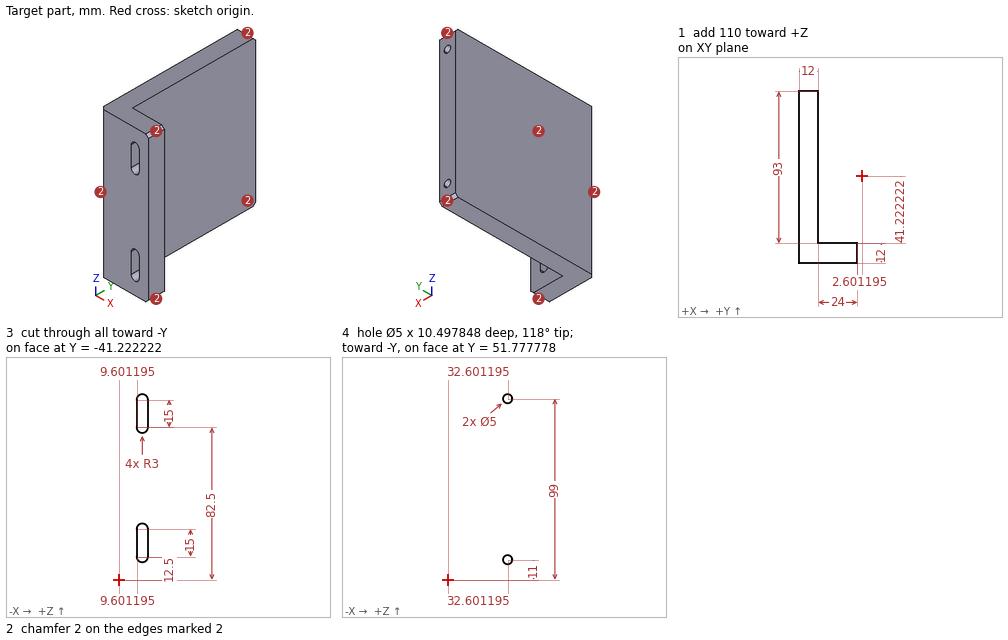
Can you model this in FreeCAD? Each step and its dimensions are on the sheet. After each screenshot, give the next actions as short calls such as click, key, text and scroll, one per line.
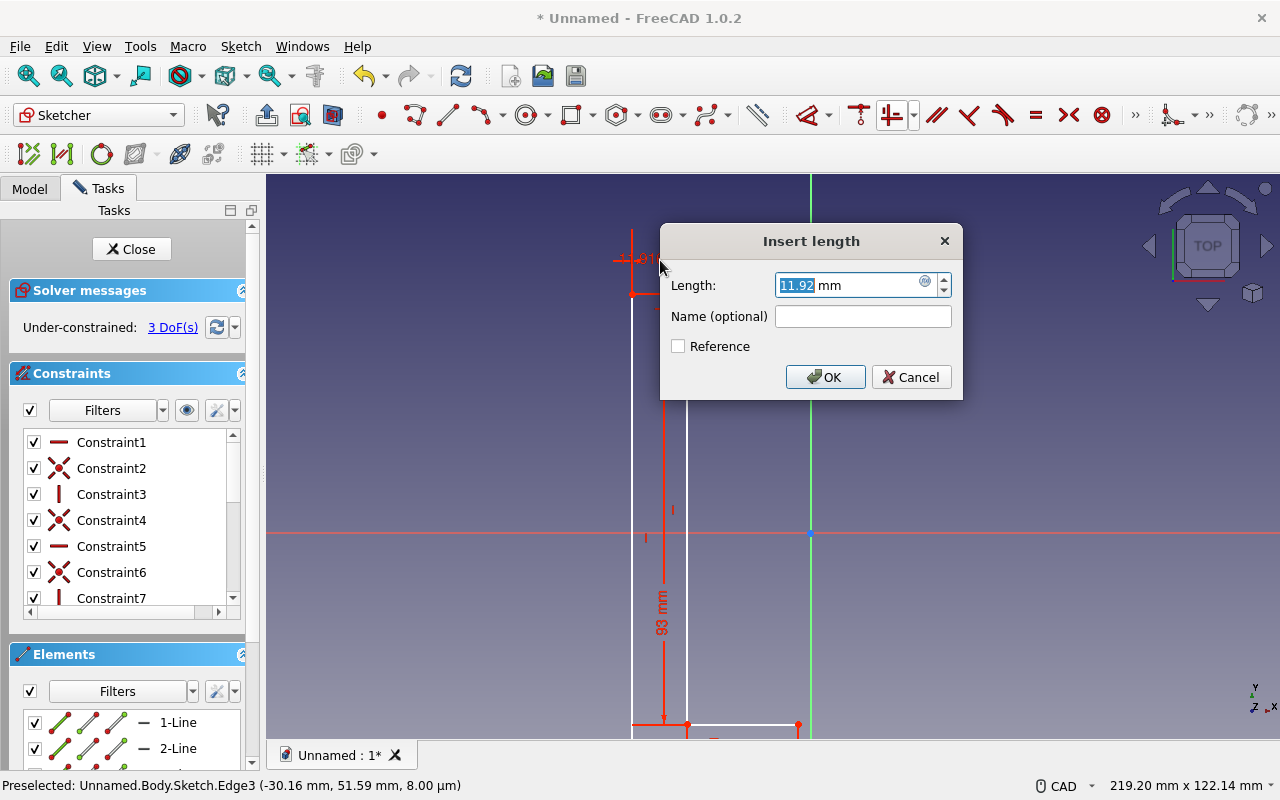
text(12)
key(Return)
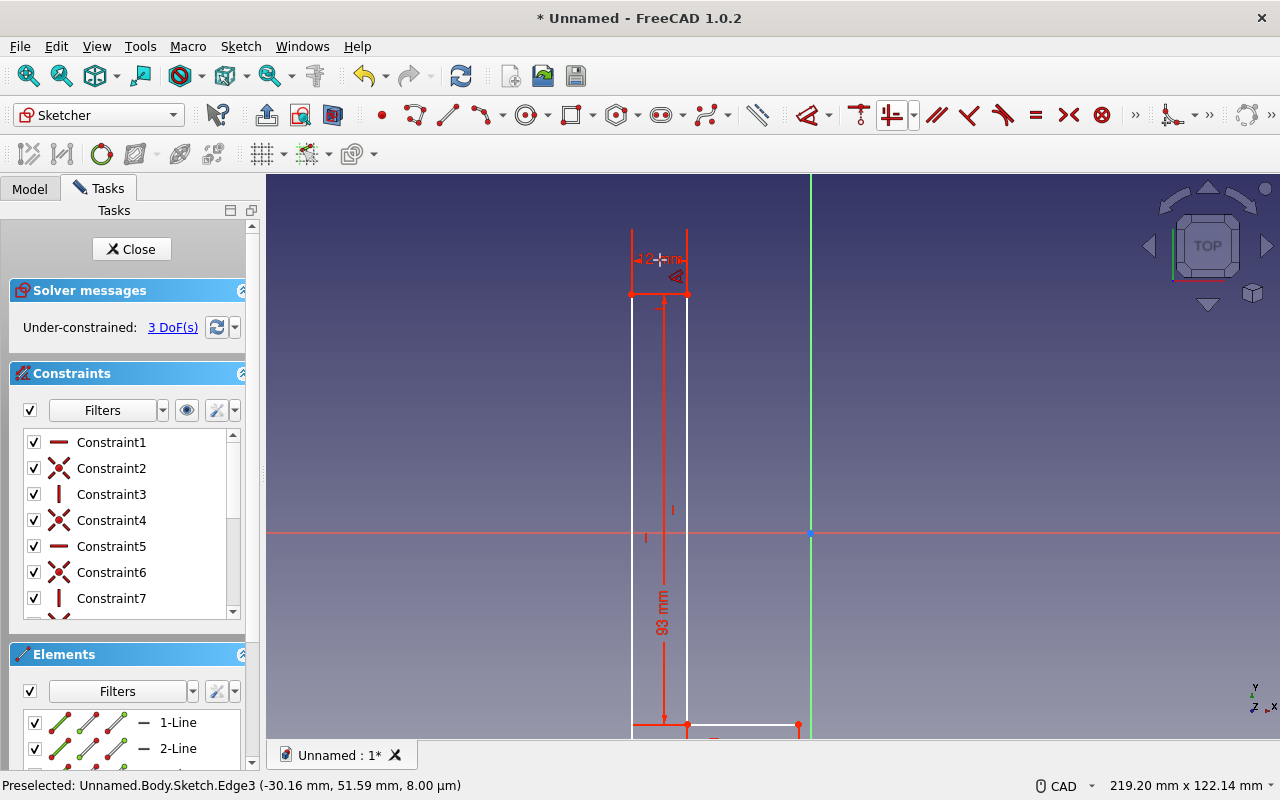
scroll(670, 294, down, 2)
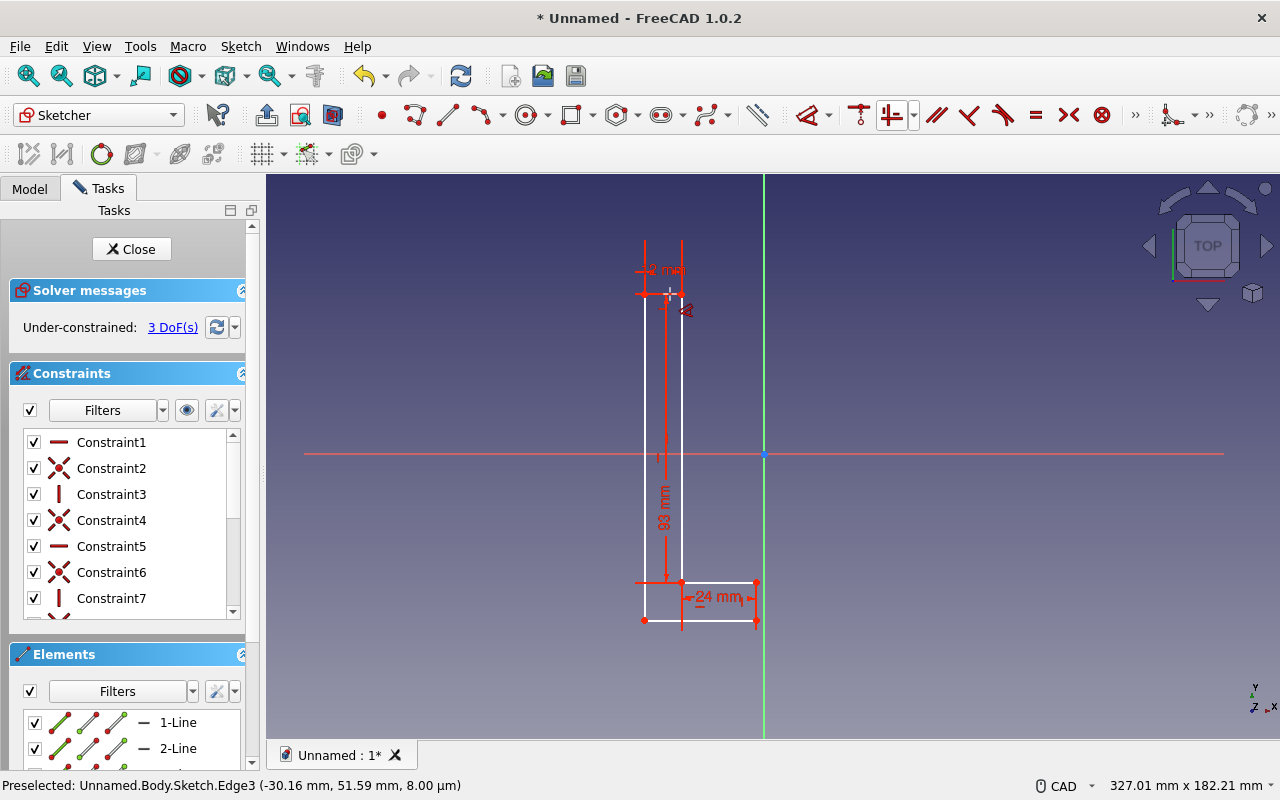
scroll(756, 609, up, 3)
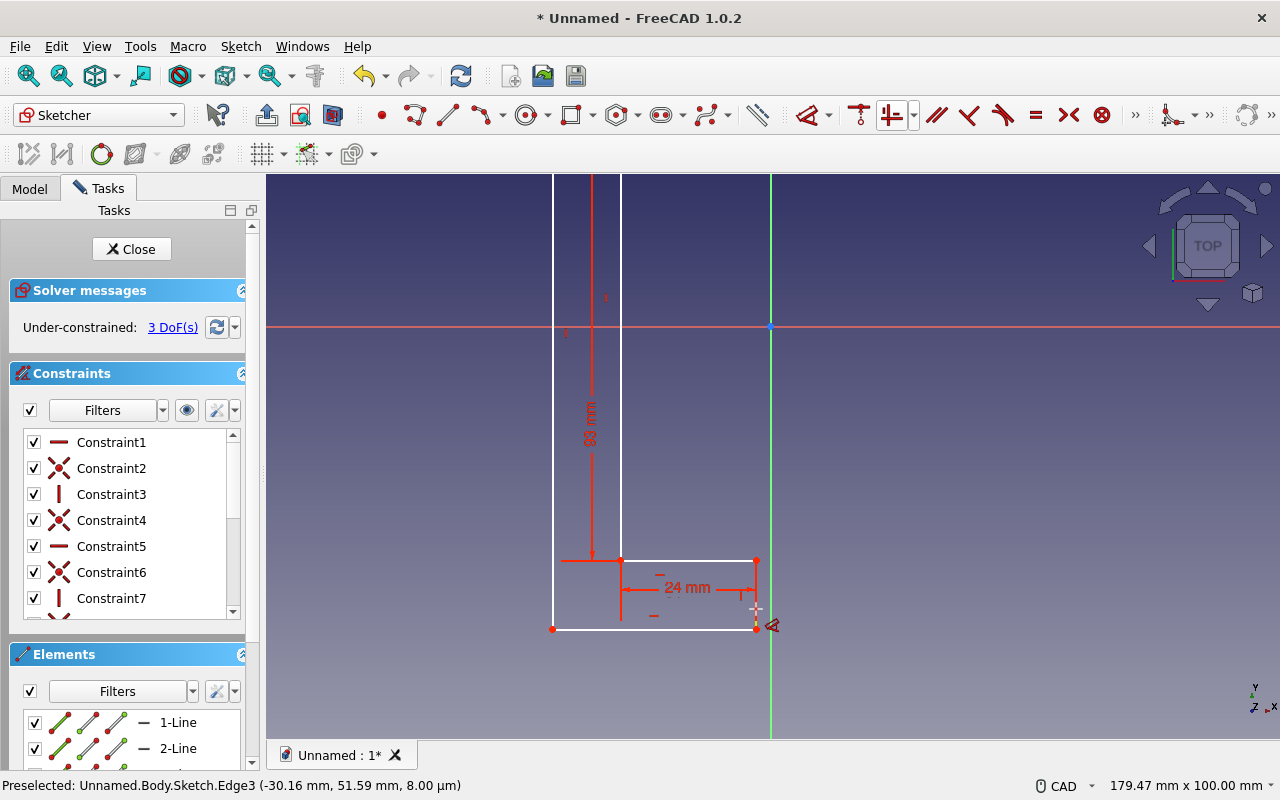
click(756, 609)
click(790, 595)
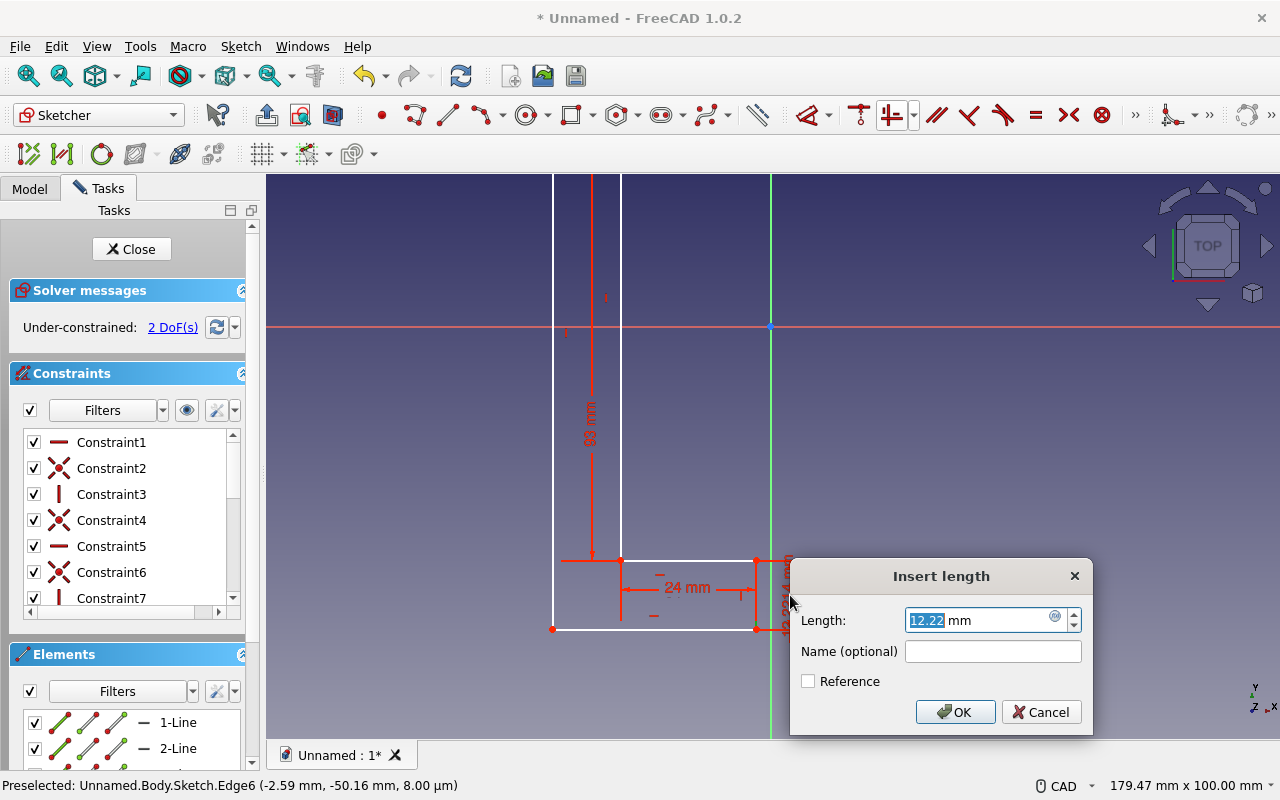
text(12)
key(Return)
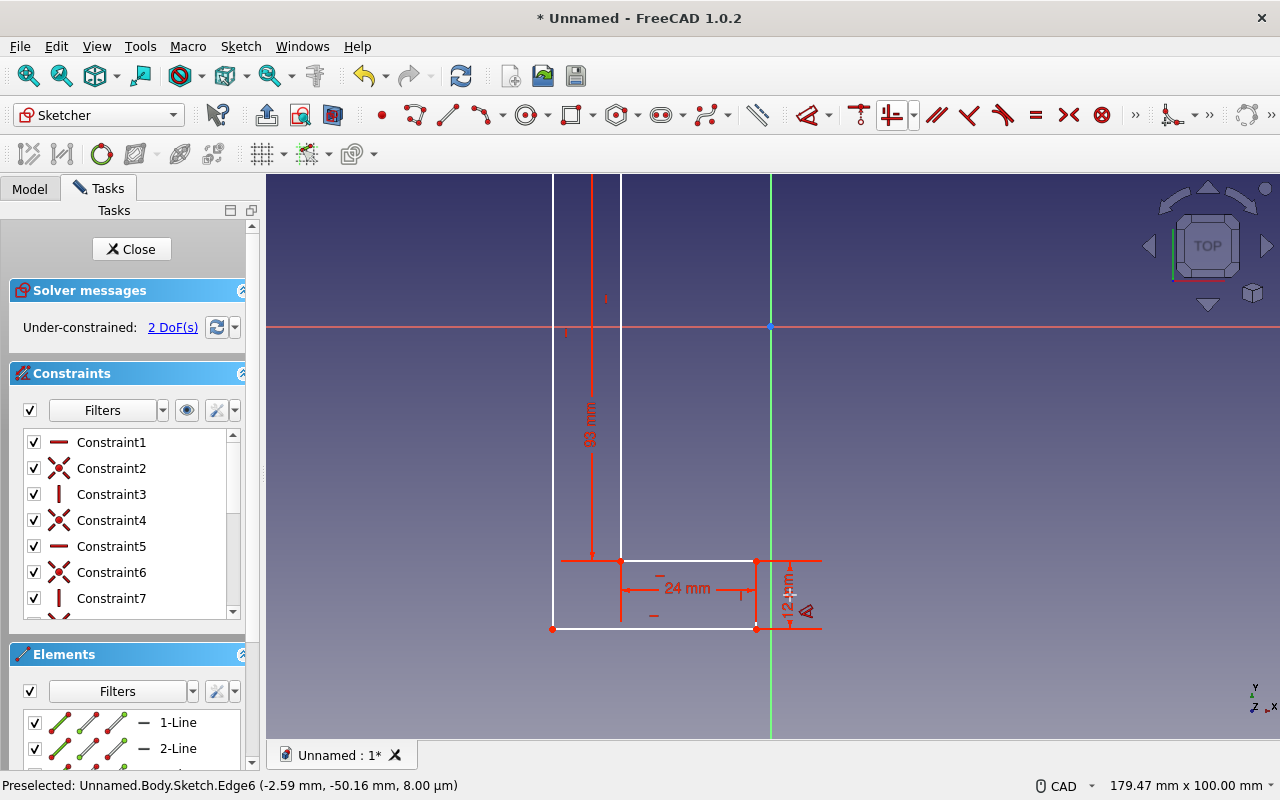
scroll(756, 561, up, 5)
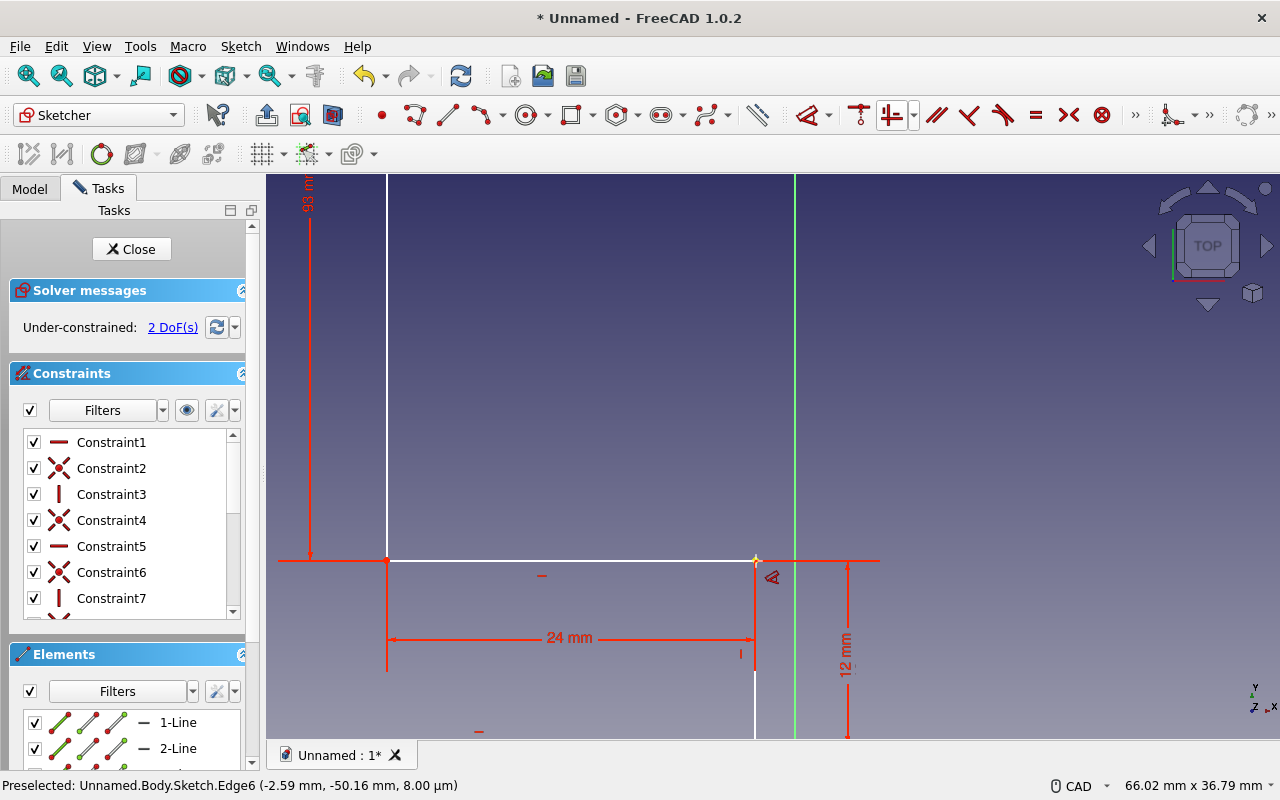
click(755, 561)
click(775, 595)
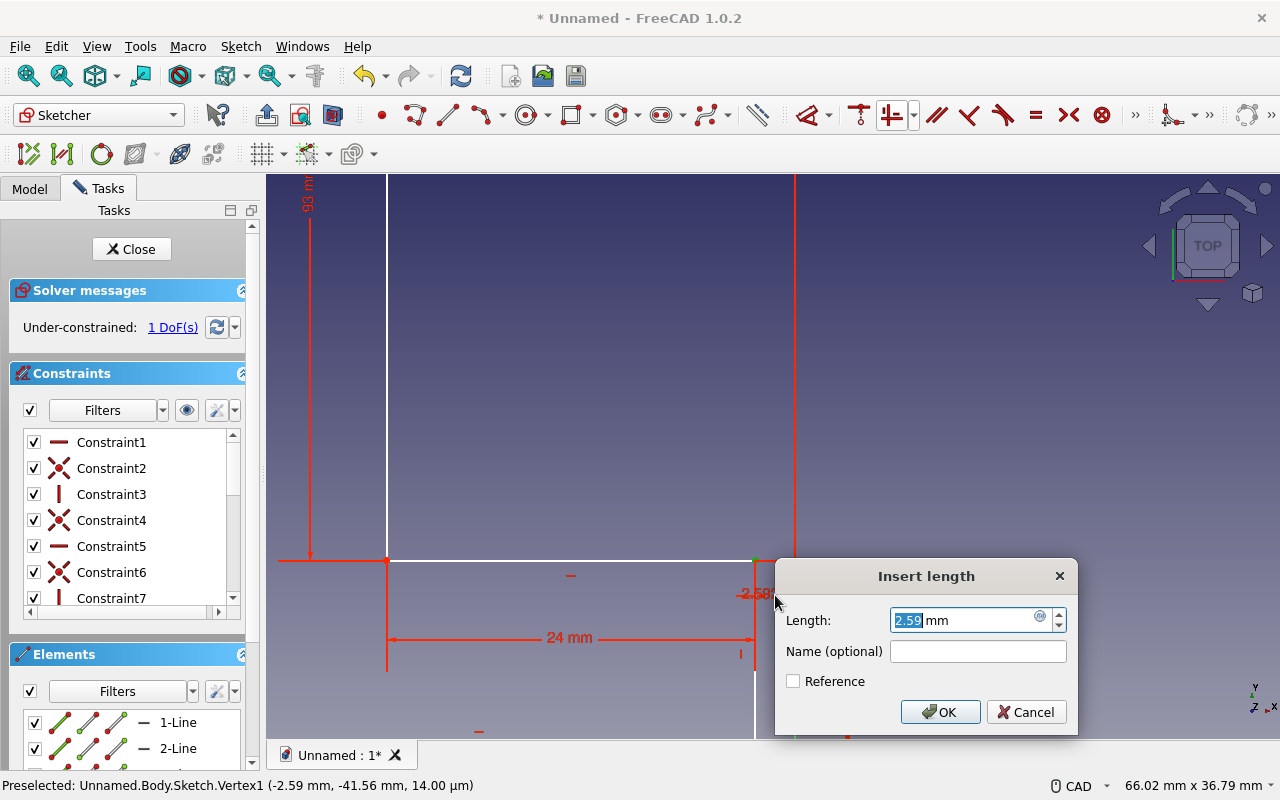
text(2.601195)
key(Return)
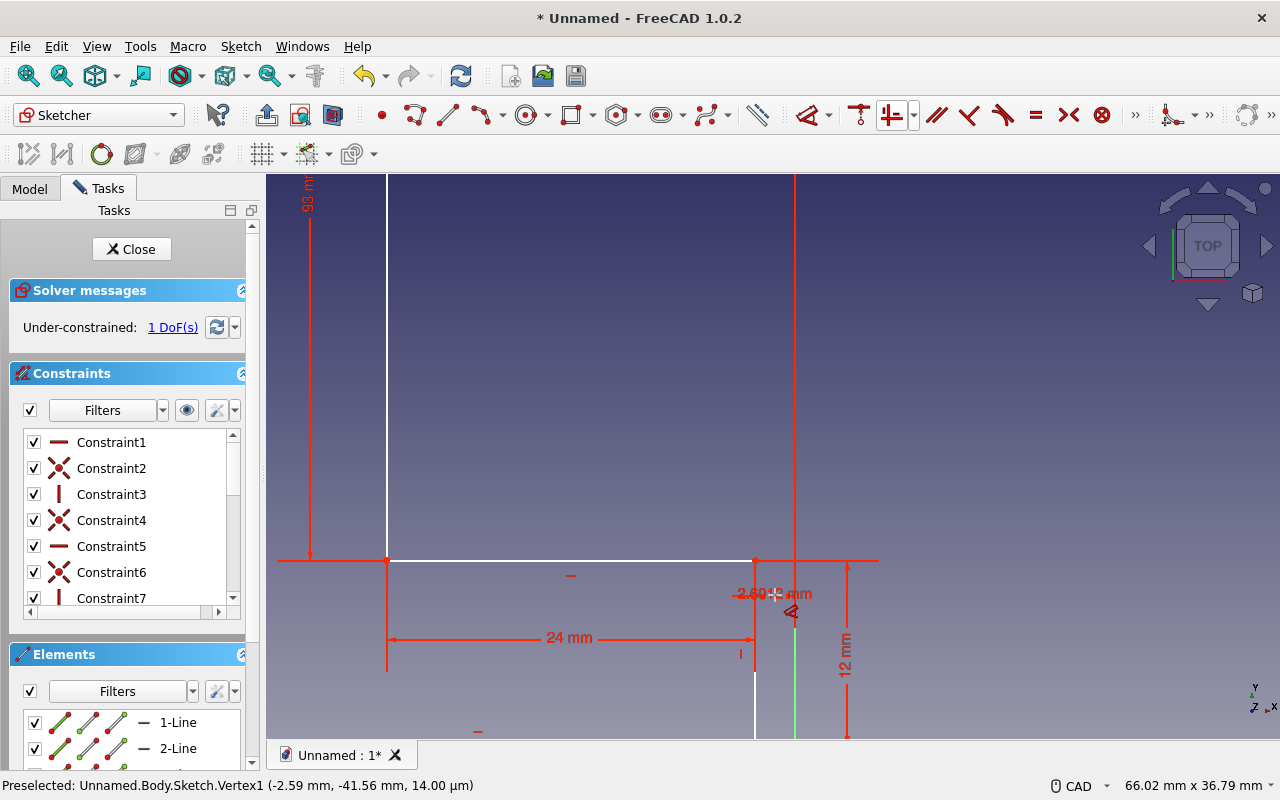
scroll(757, 589, down, 8)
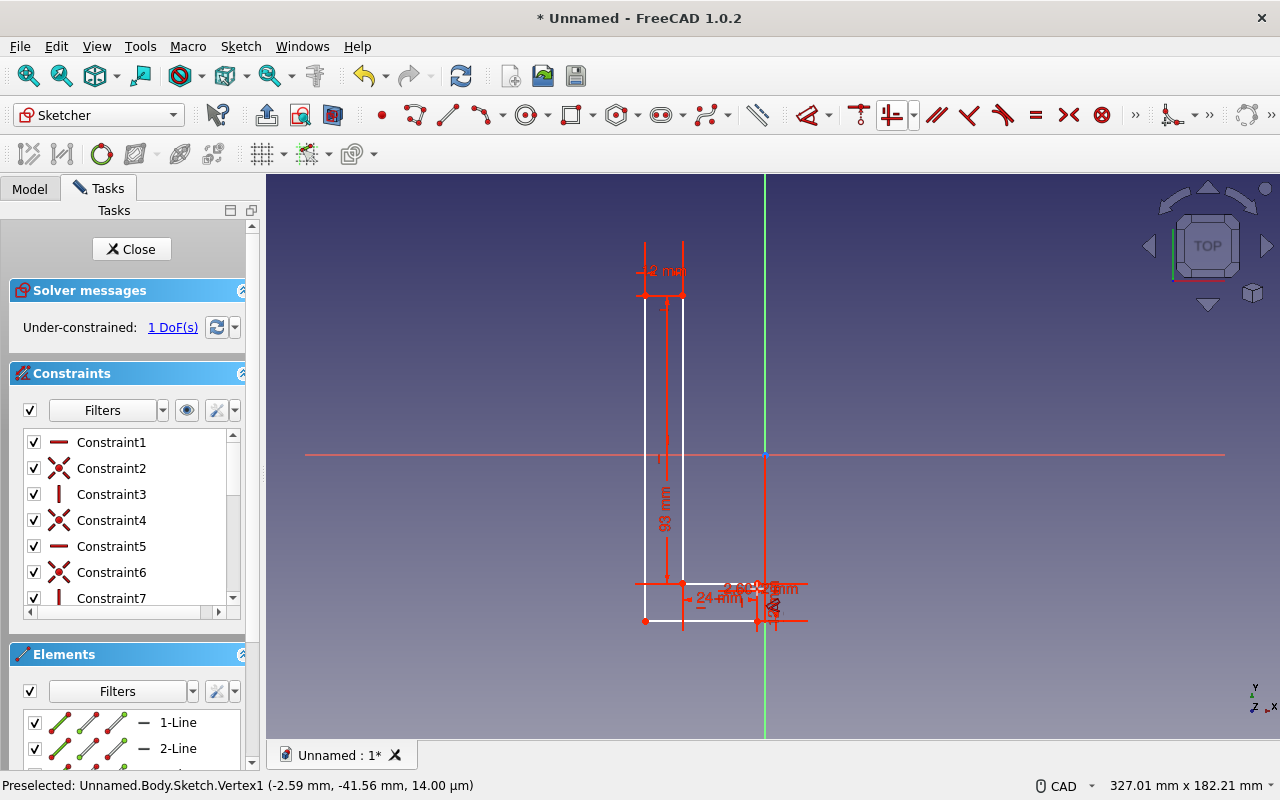
click(757, 584)
click(799, 519)